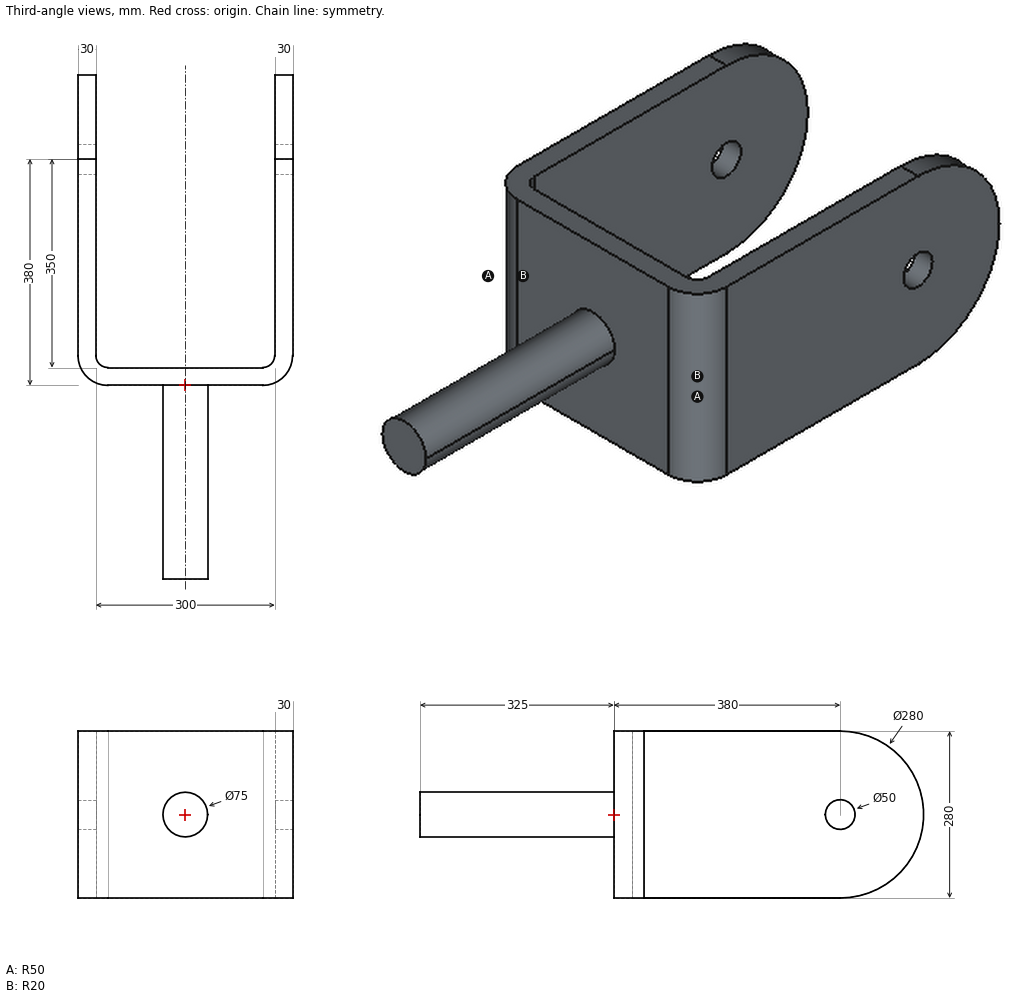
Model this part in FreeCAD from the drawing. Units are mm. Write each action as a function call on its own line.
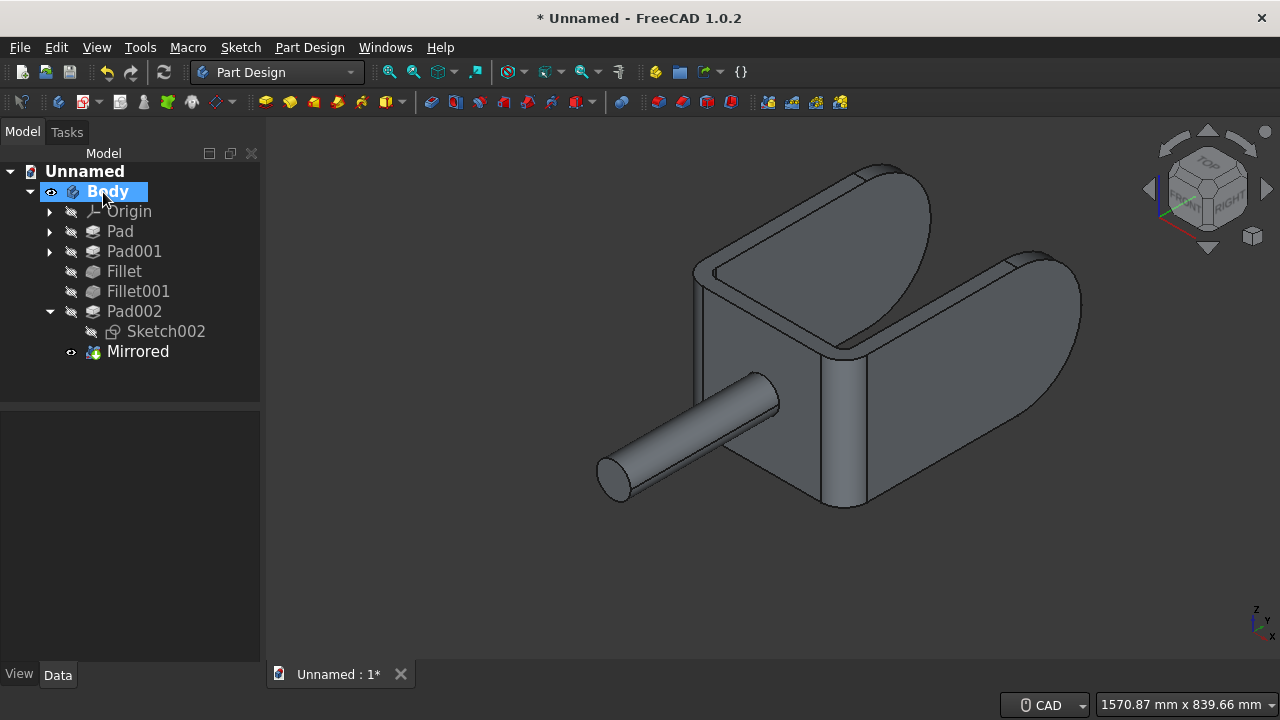
key(6)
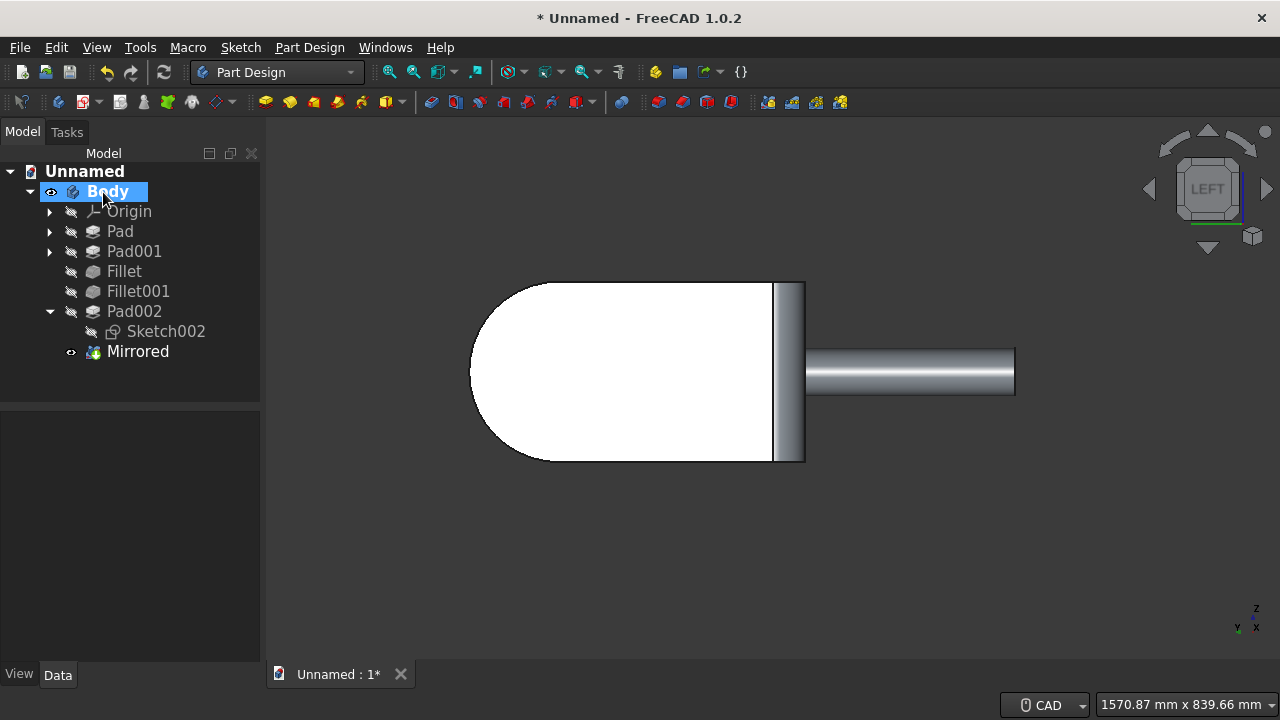
click(578, 371)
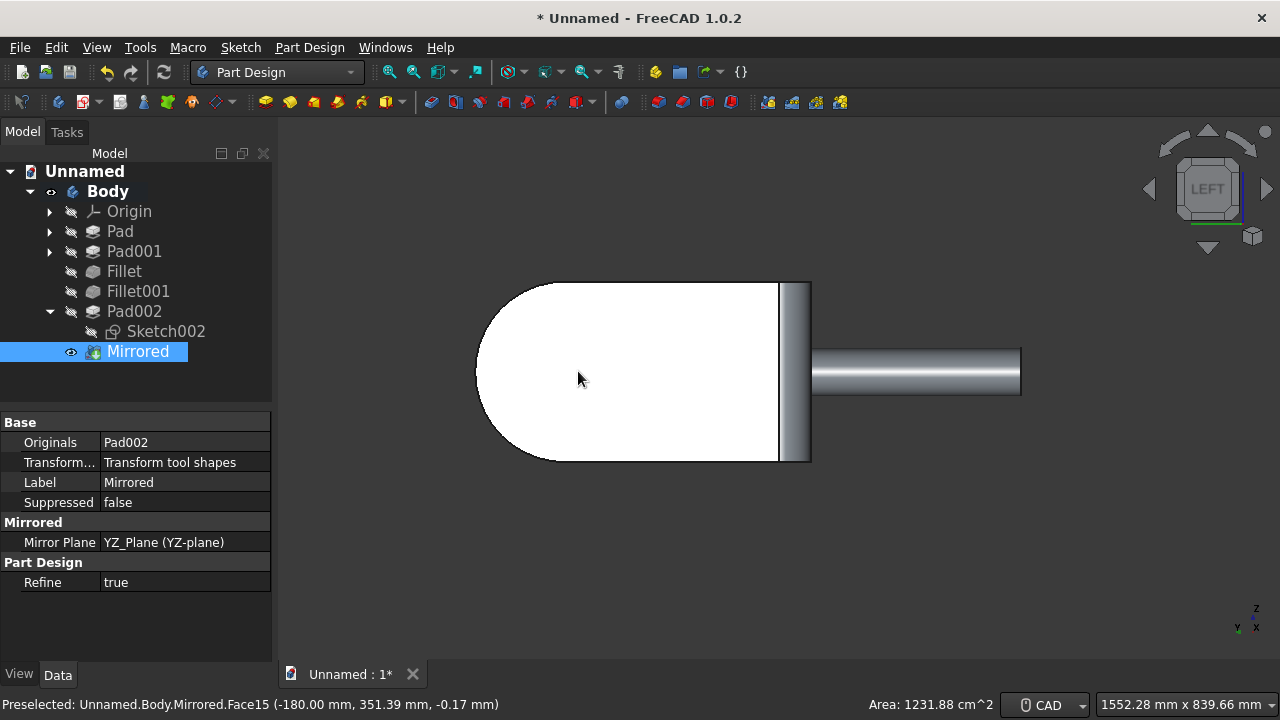
click(84, 102)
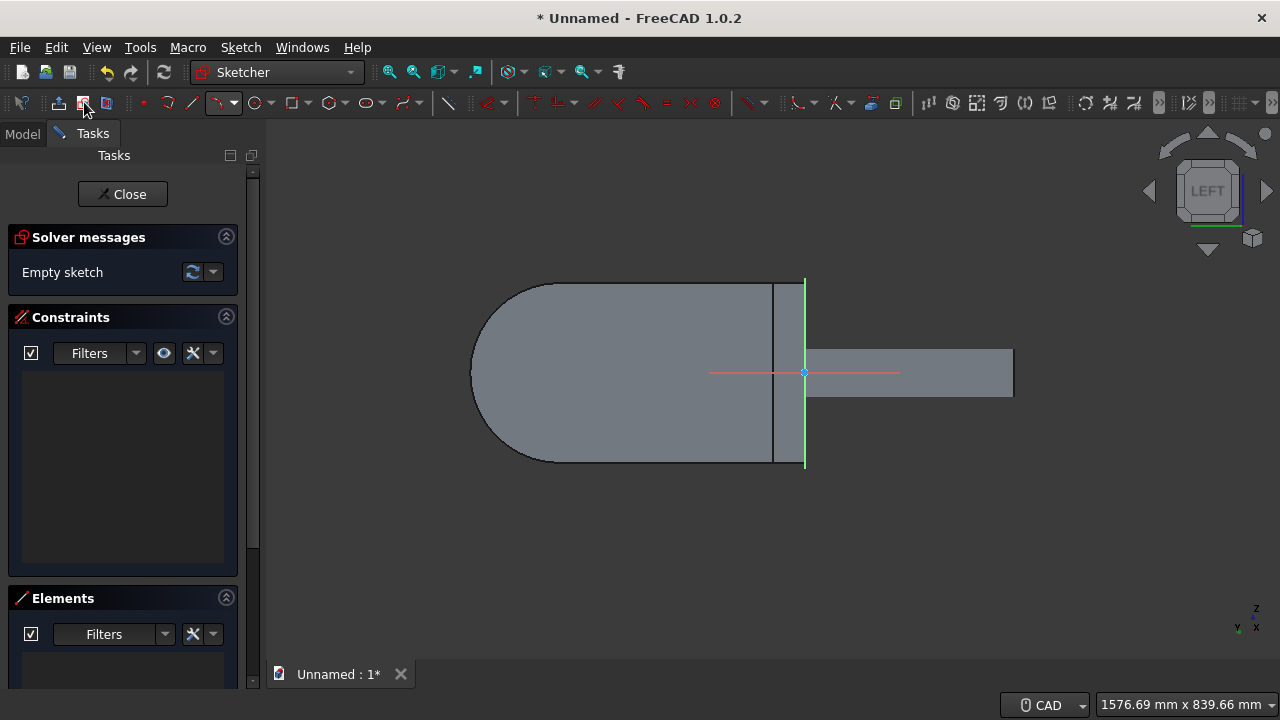
scroll(546, 371, up, 12)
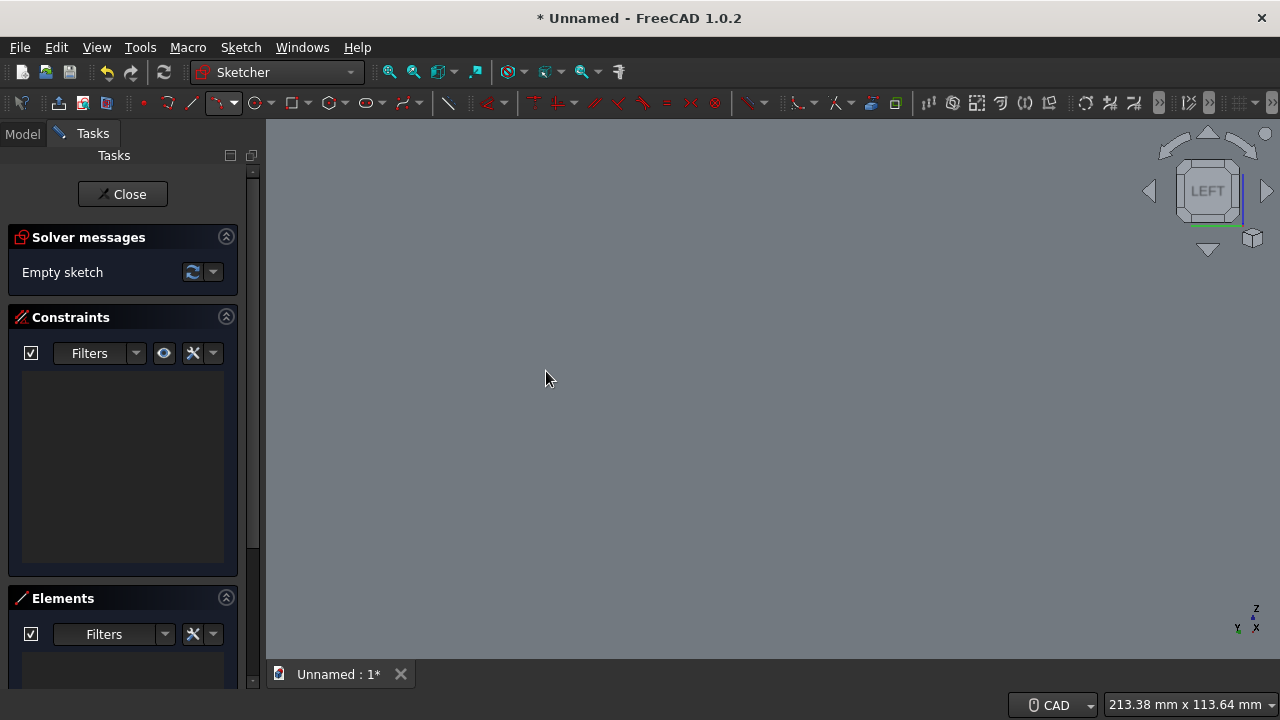
click(256, 104)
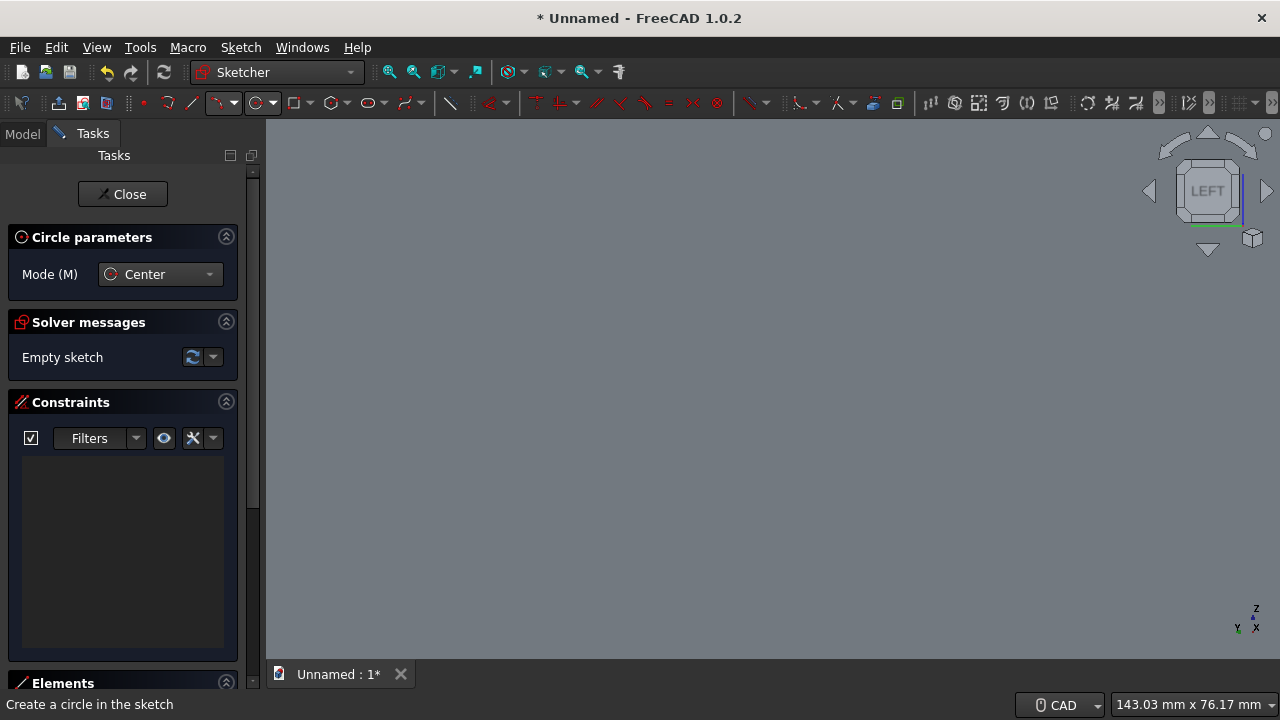
click(701, 388)
move(826, 262)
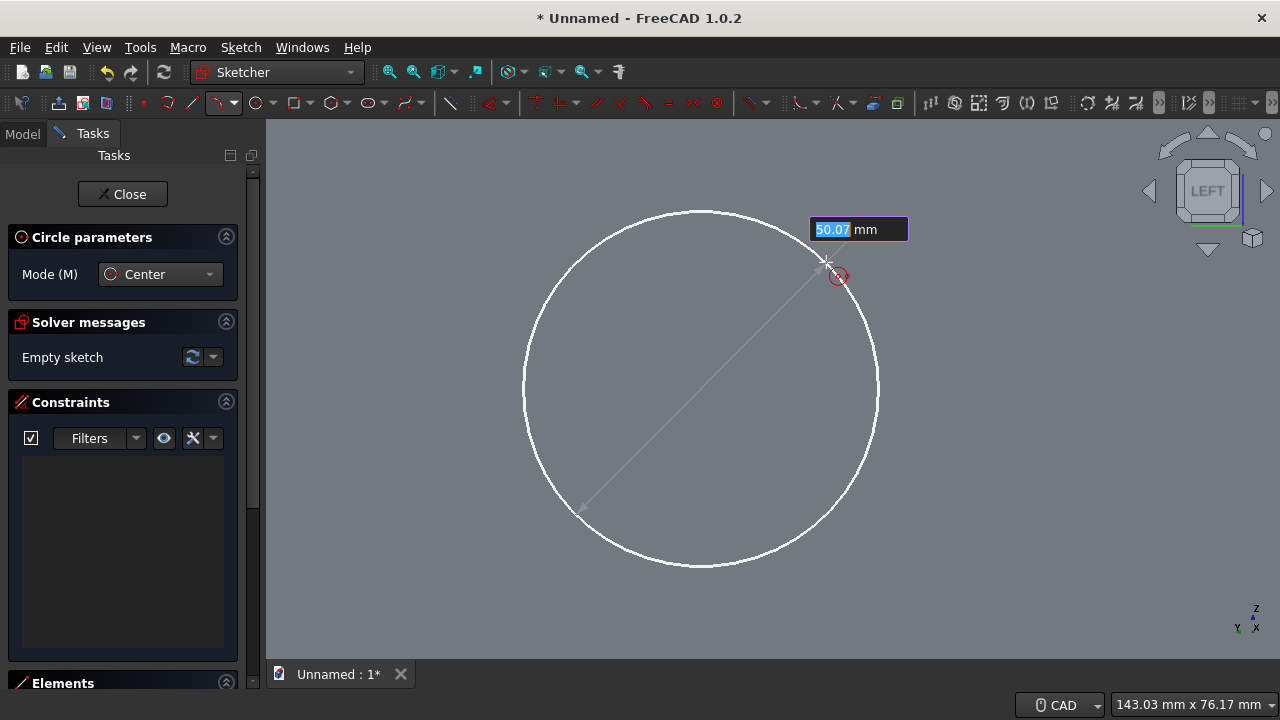
text(50)
key(Return)
key(Escape)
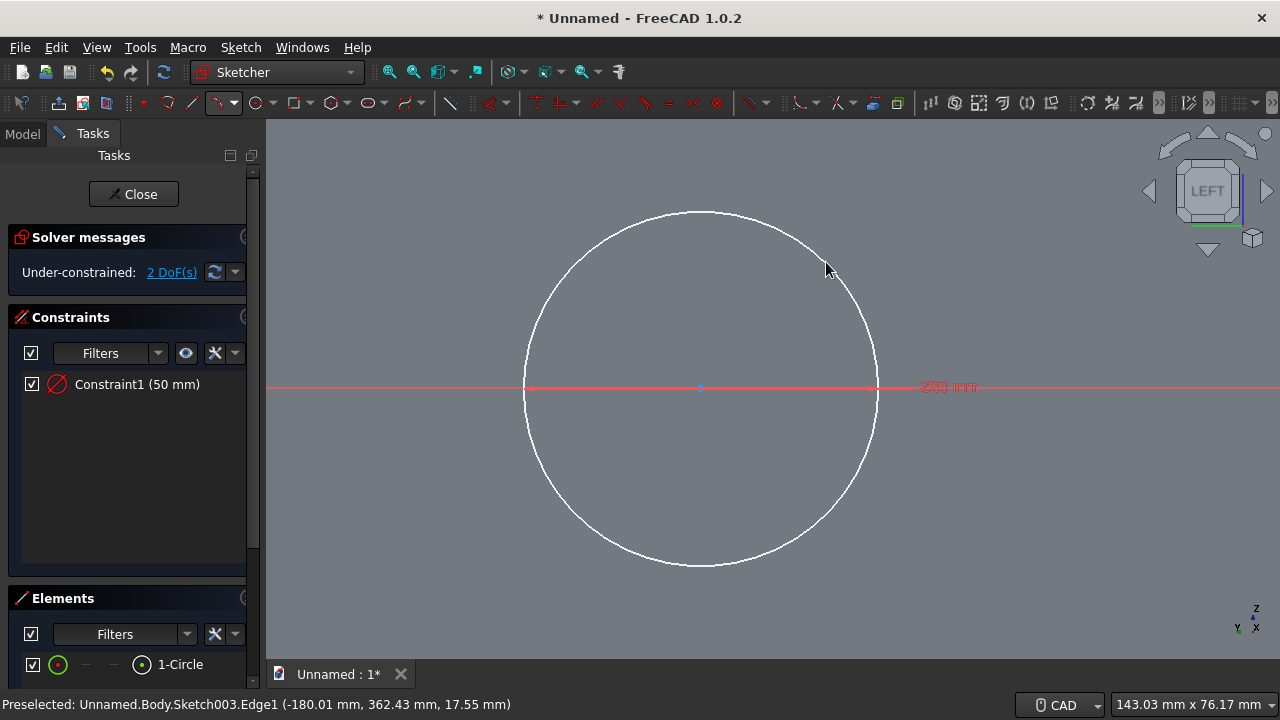
click(701, 389)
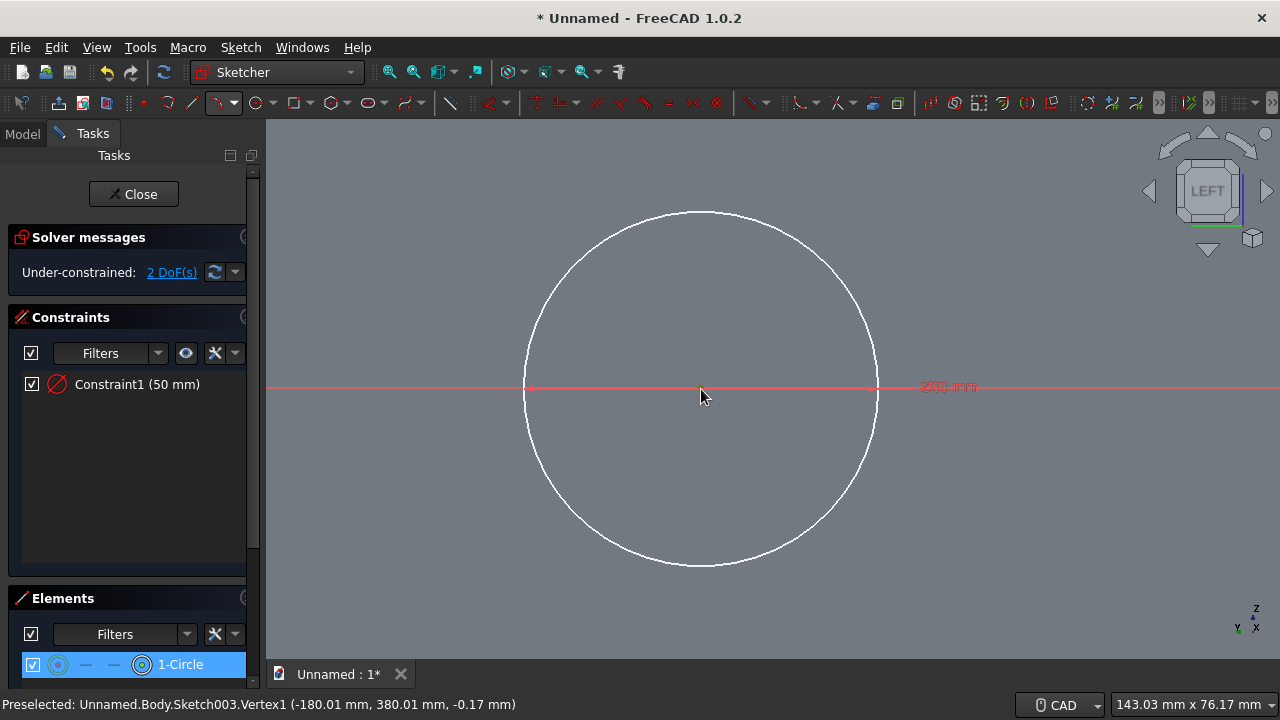
click(353, 388)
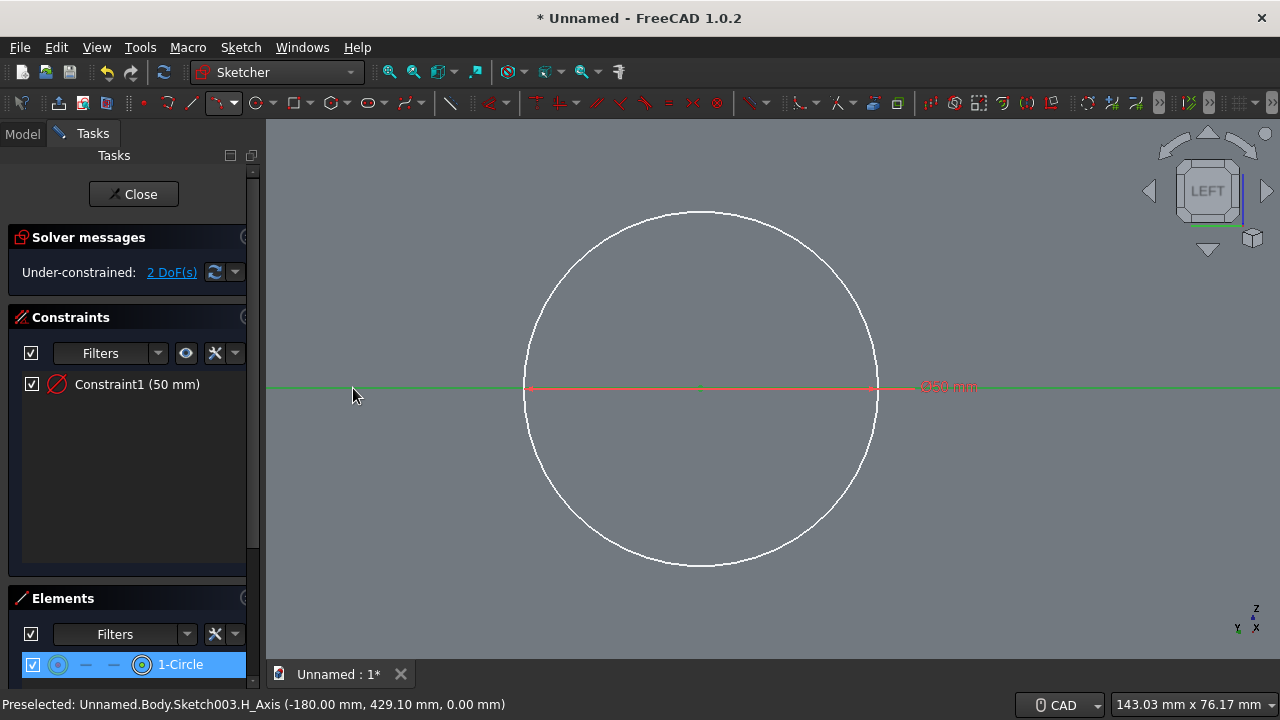
click(536, 104)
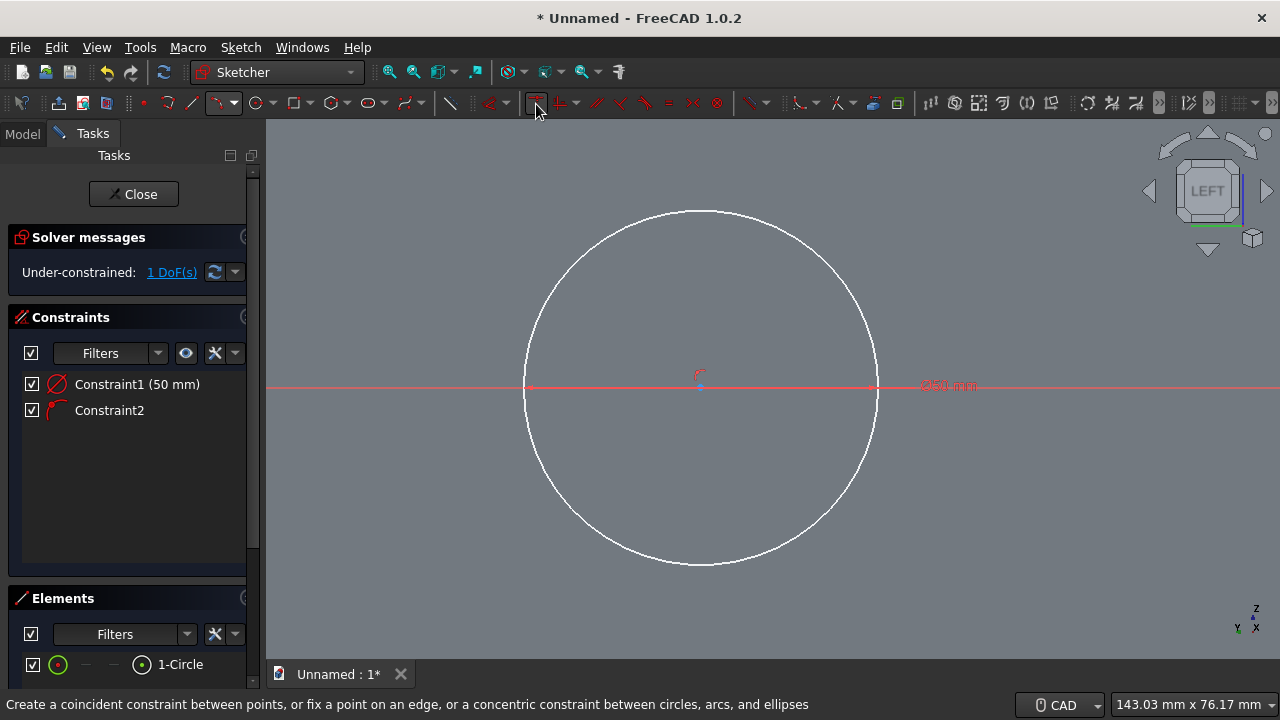
click(490, 104)